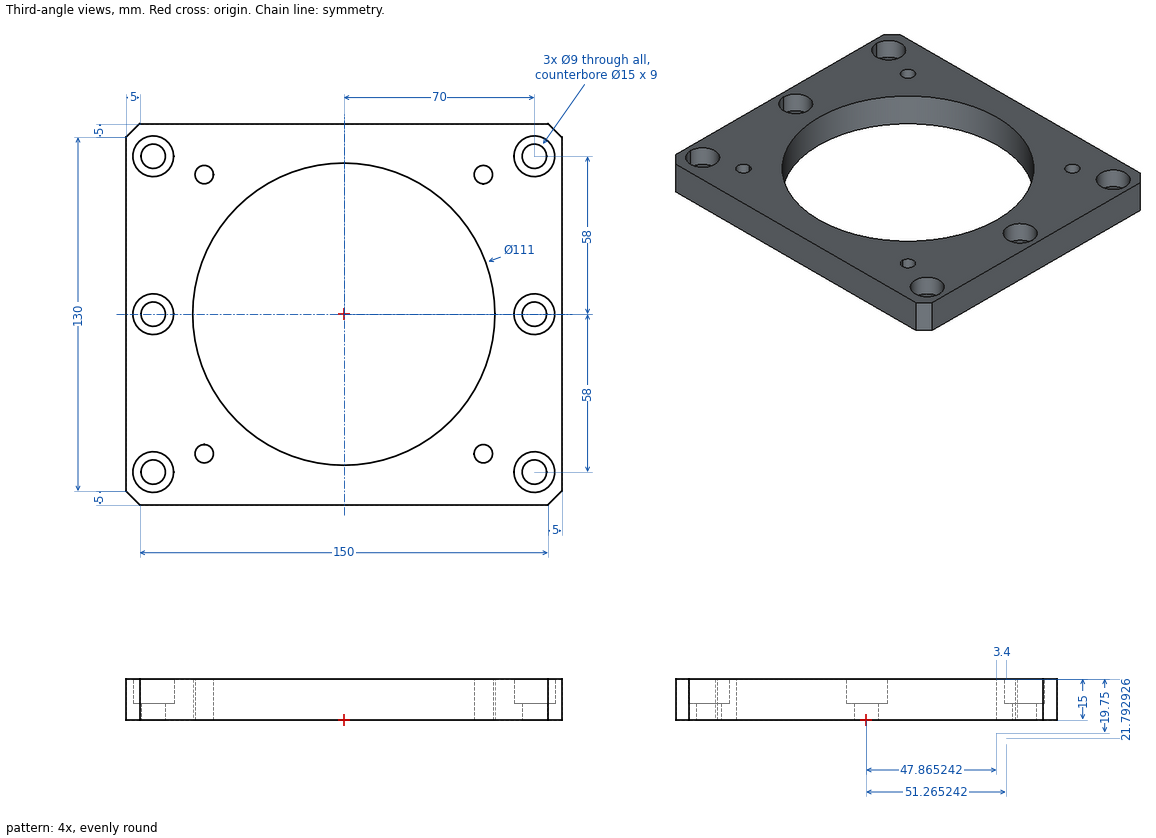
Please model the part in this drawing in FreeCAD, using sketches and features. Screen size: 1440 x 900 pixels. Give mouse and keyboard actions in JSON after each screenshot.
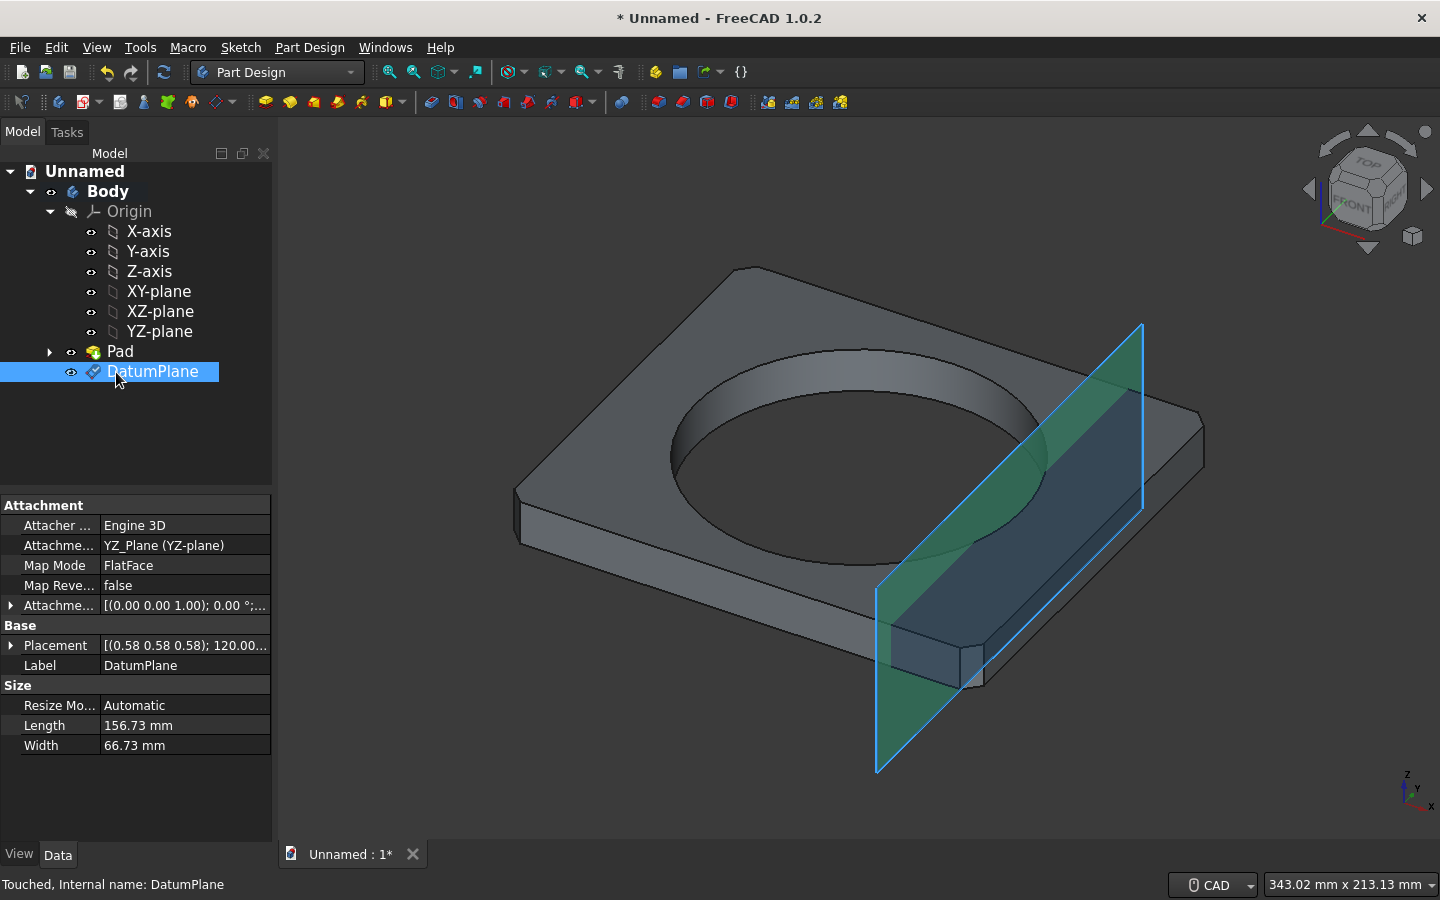
{"action": "left_click", "coordinate": [84, 102]}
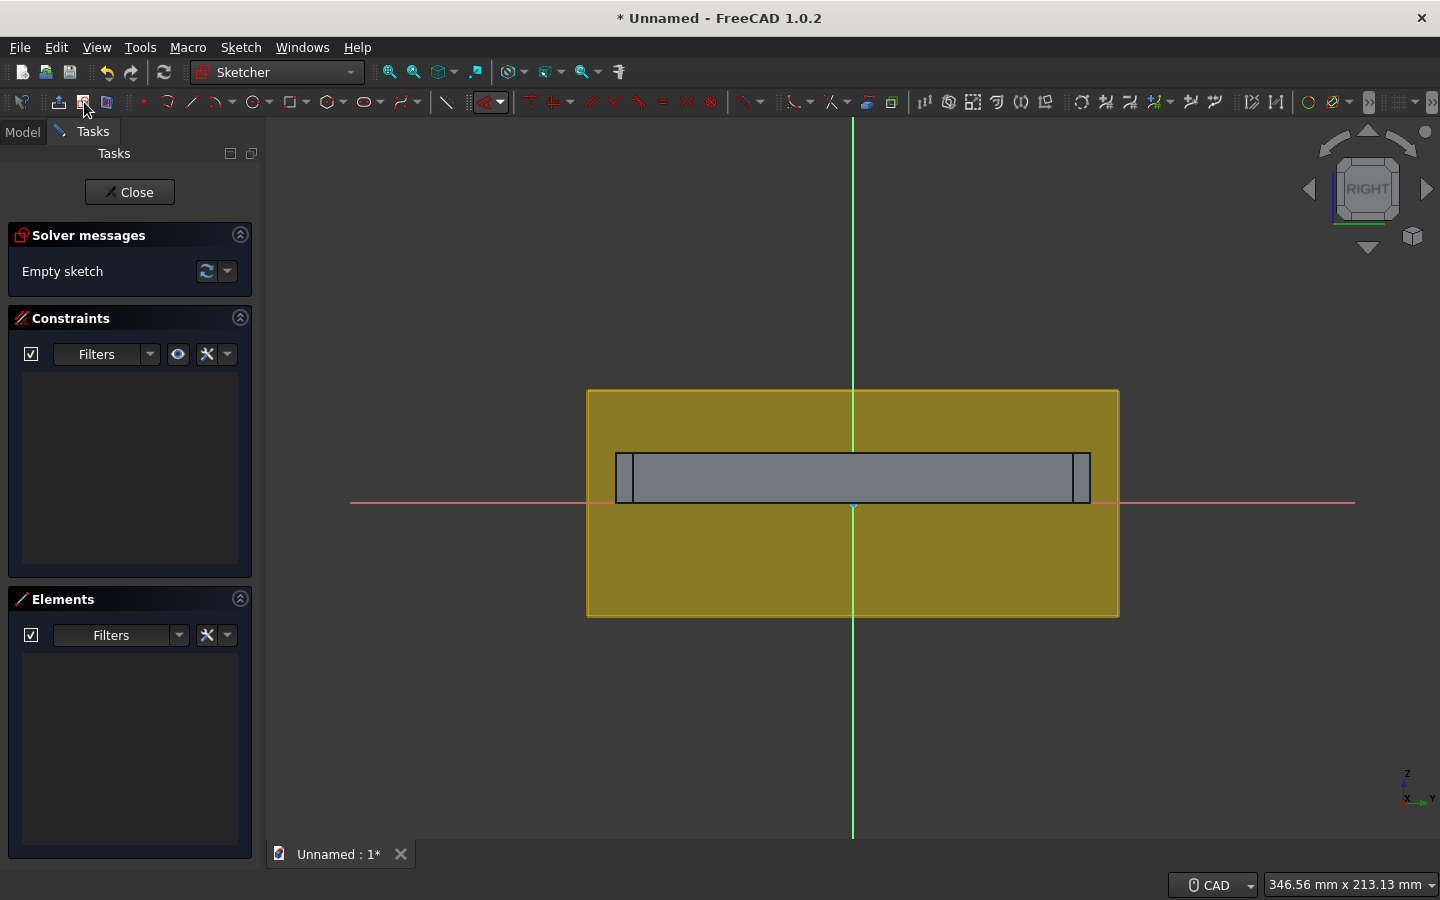
{"action": "left_click", "coordinate": [108, 102]}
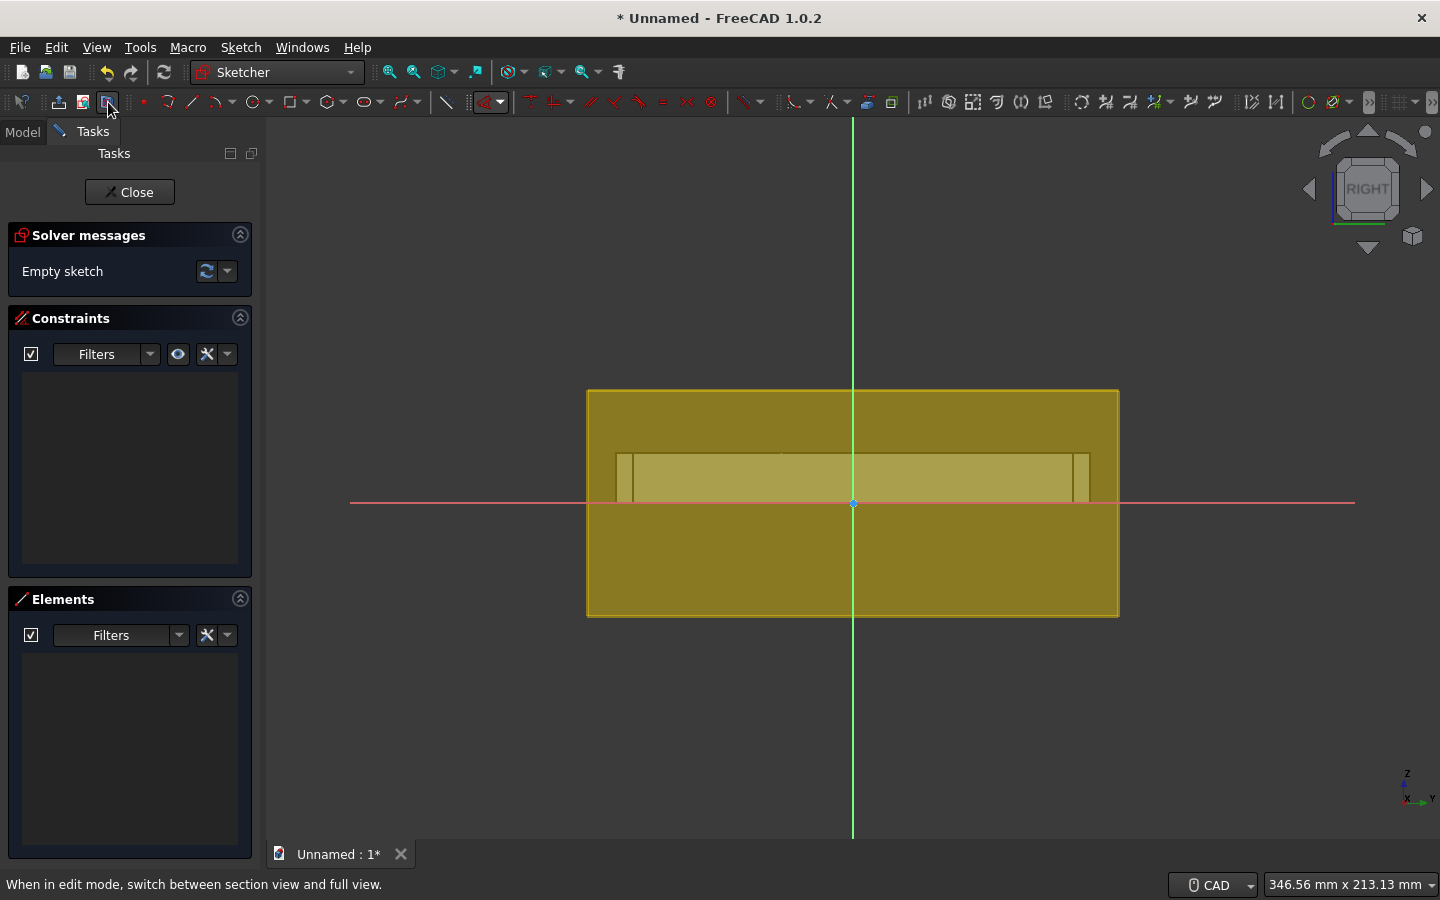
{"action": "scroll", "coordinate": [991, 513], "scroll_direction": "up", "scroll_amount": 7}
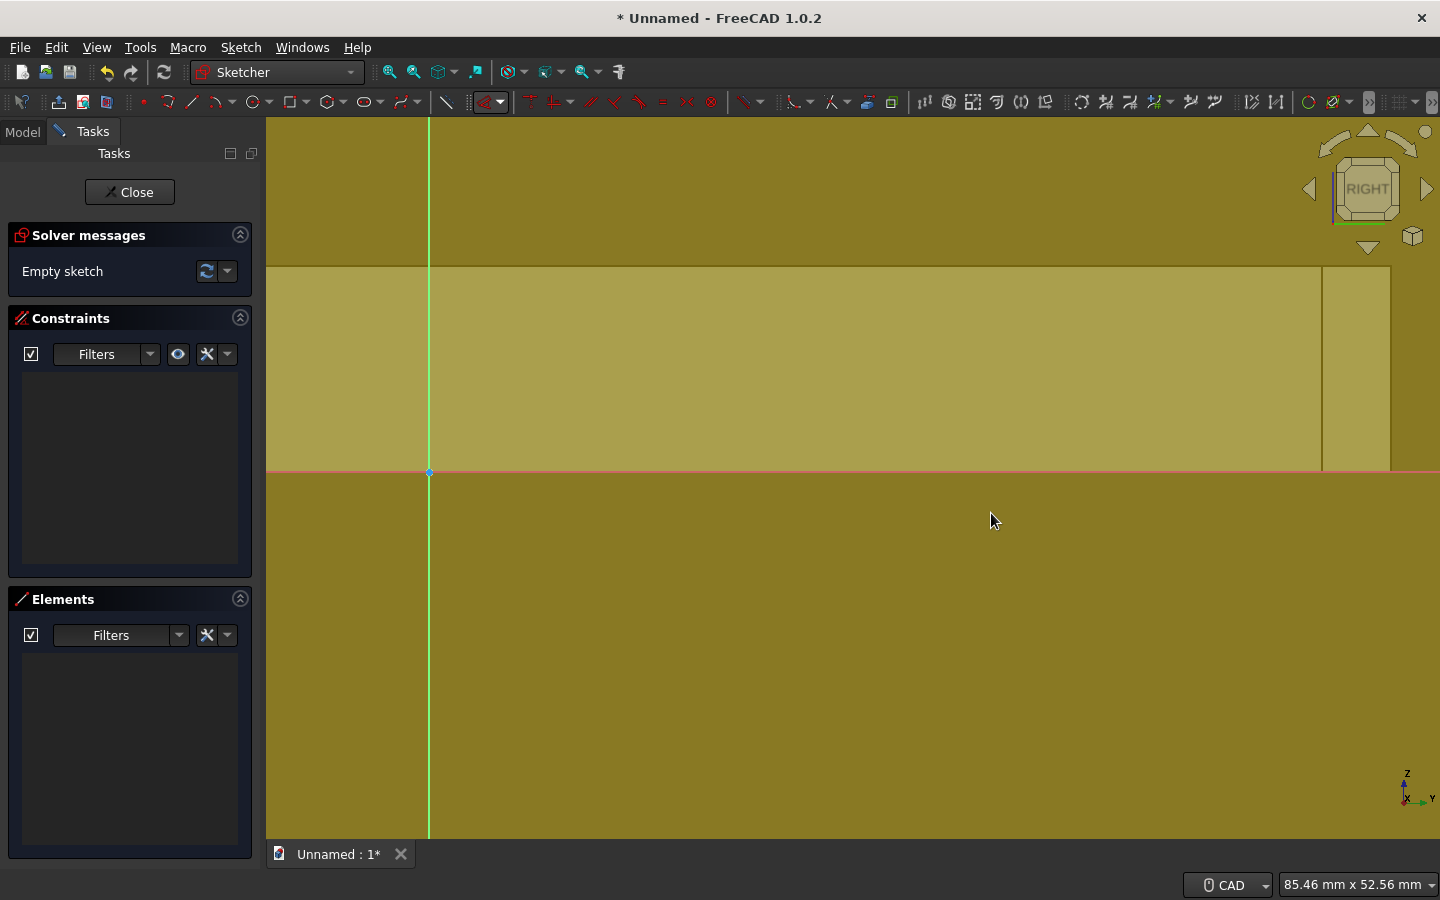
{"action": "left_click", "coordinate": [168, 102]}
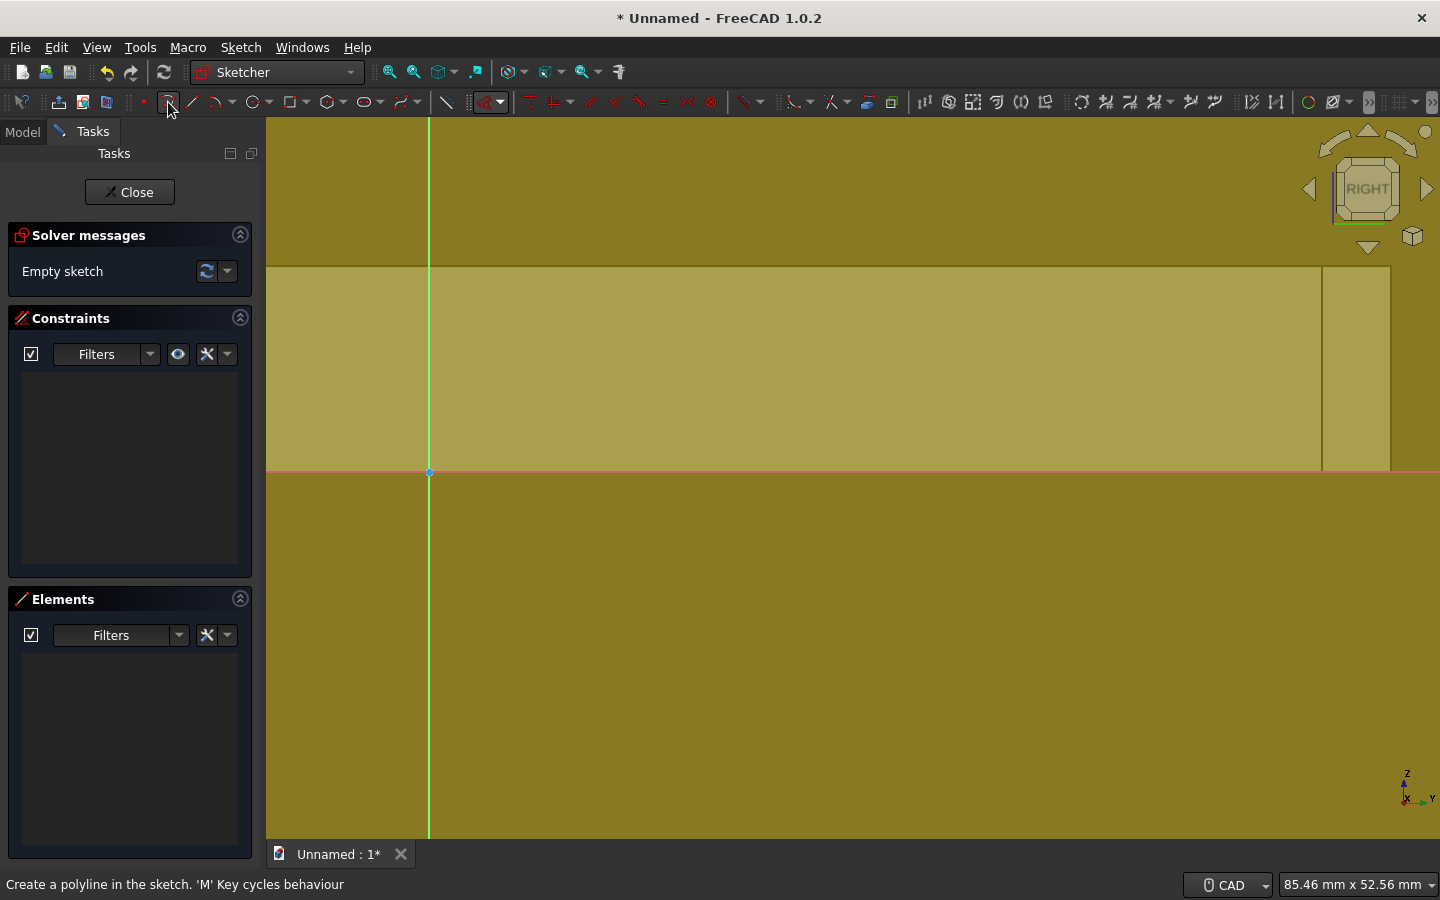
{"action": "left_click", "coordinate": [1087, 538]}
{"action": "left_click", "coordinate": [1134, 566]}
{"action": "left_click", "coordinate": [1134, 266]}
{"action": "left_click", "coordinate": [1087, 266]}
{"action": "left_click", "coordinate": [1087, 539]}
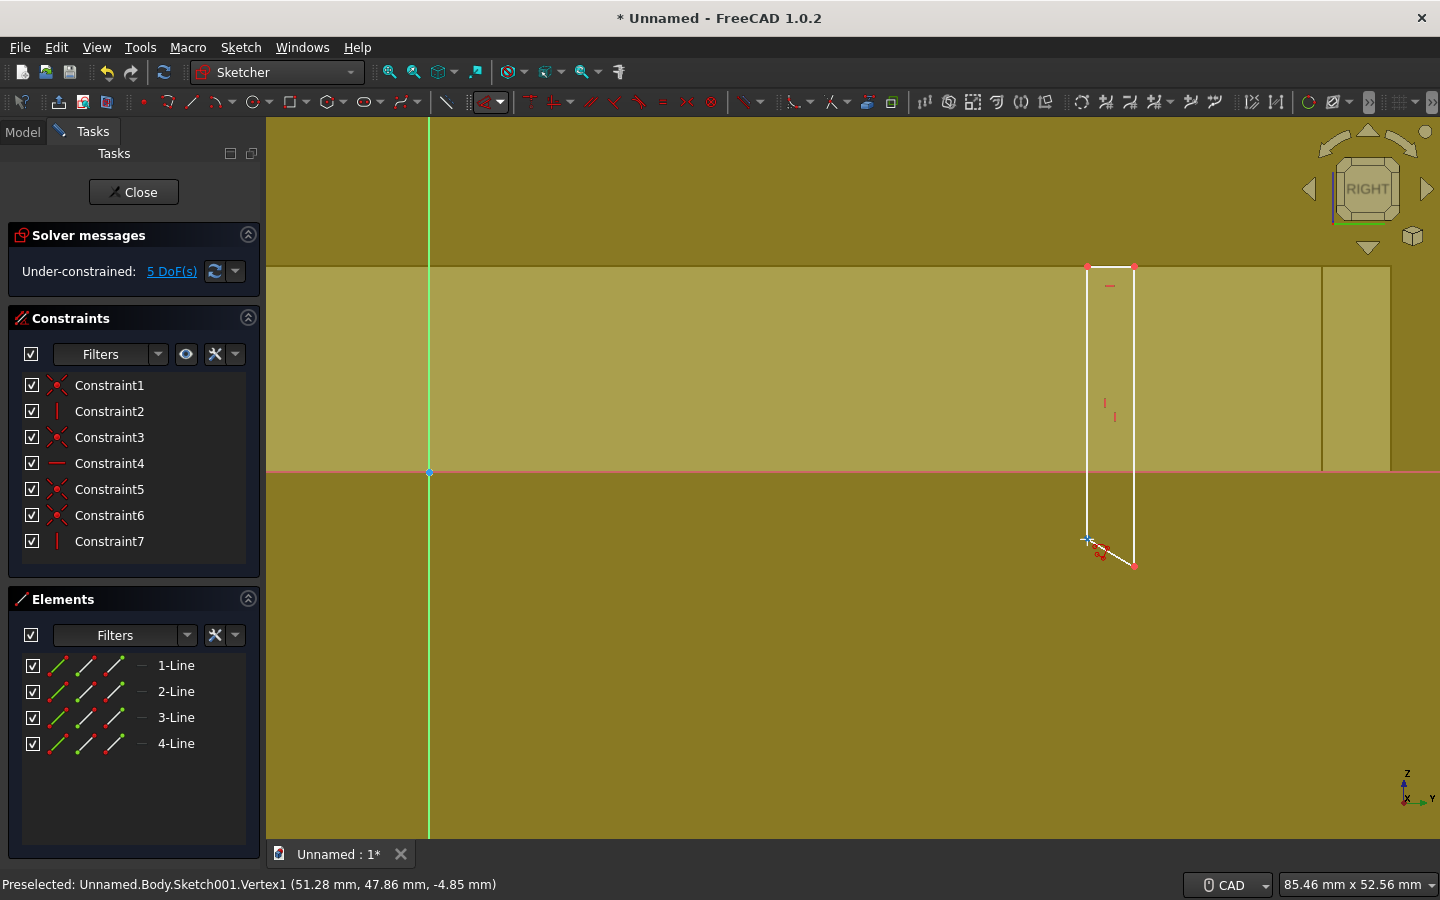
{"action": "left_click", "coordinate": [192, 102]}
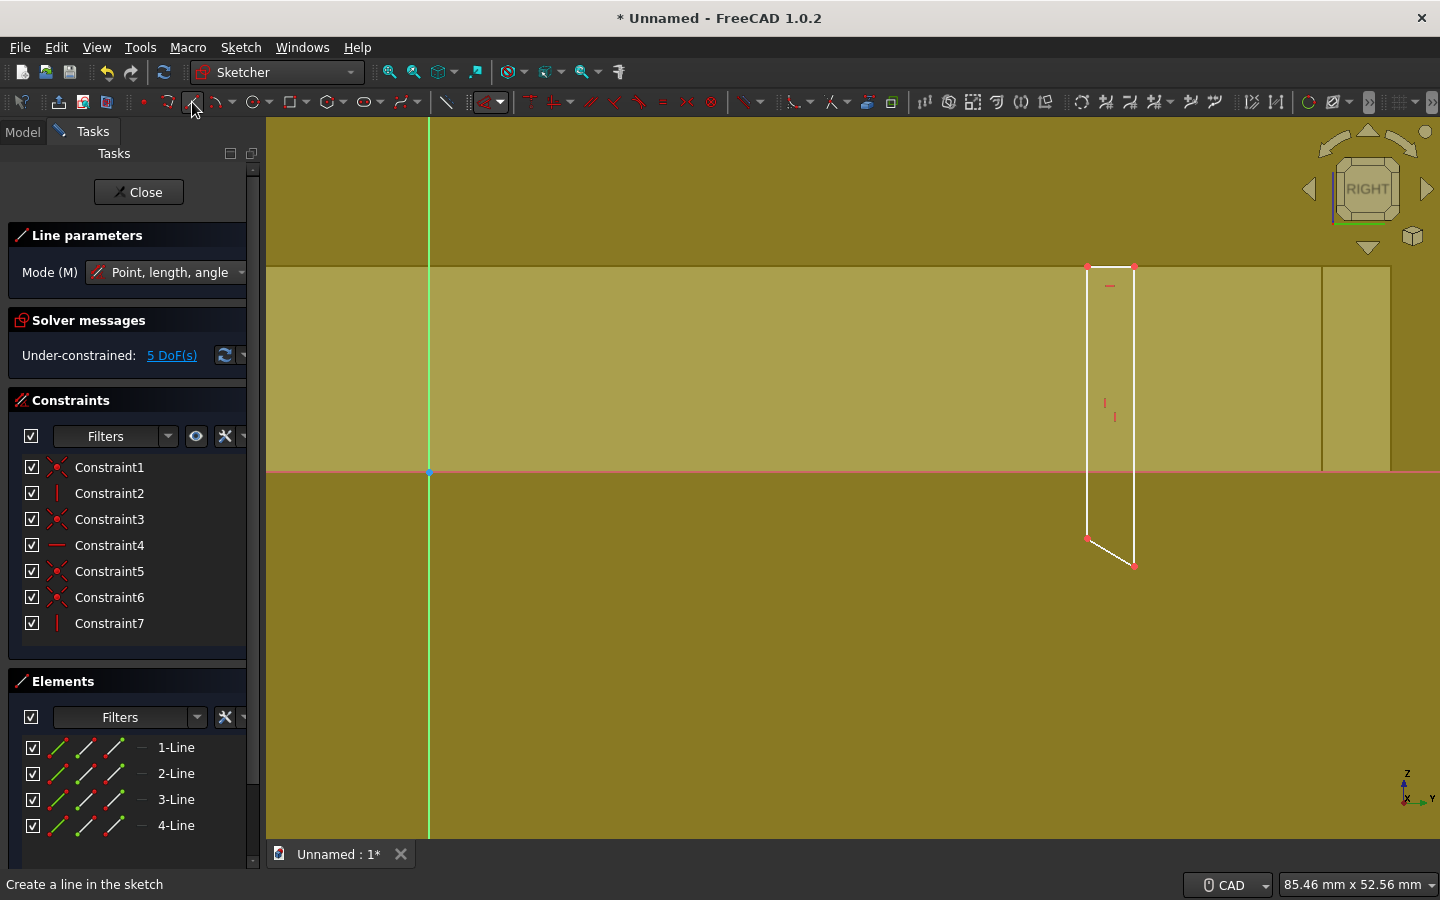
{"action": "left_click", "coordinate": [1134, 596]}
{"action": "left_click", "coordinate": [1134, 685]}
{"action": "key", "text": "Escape"}